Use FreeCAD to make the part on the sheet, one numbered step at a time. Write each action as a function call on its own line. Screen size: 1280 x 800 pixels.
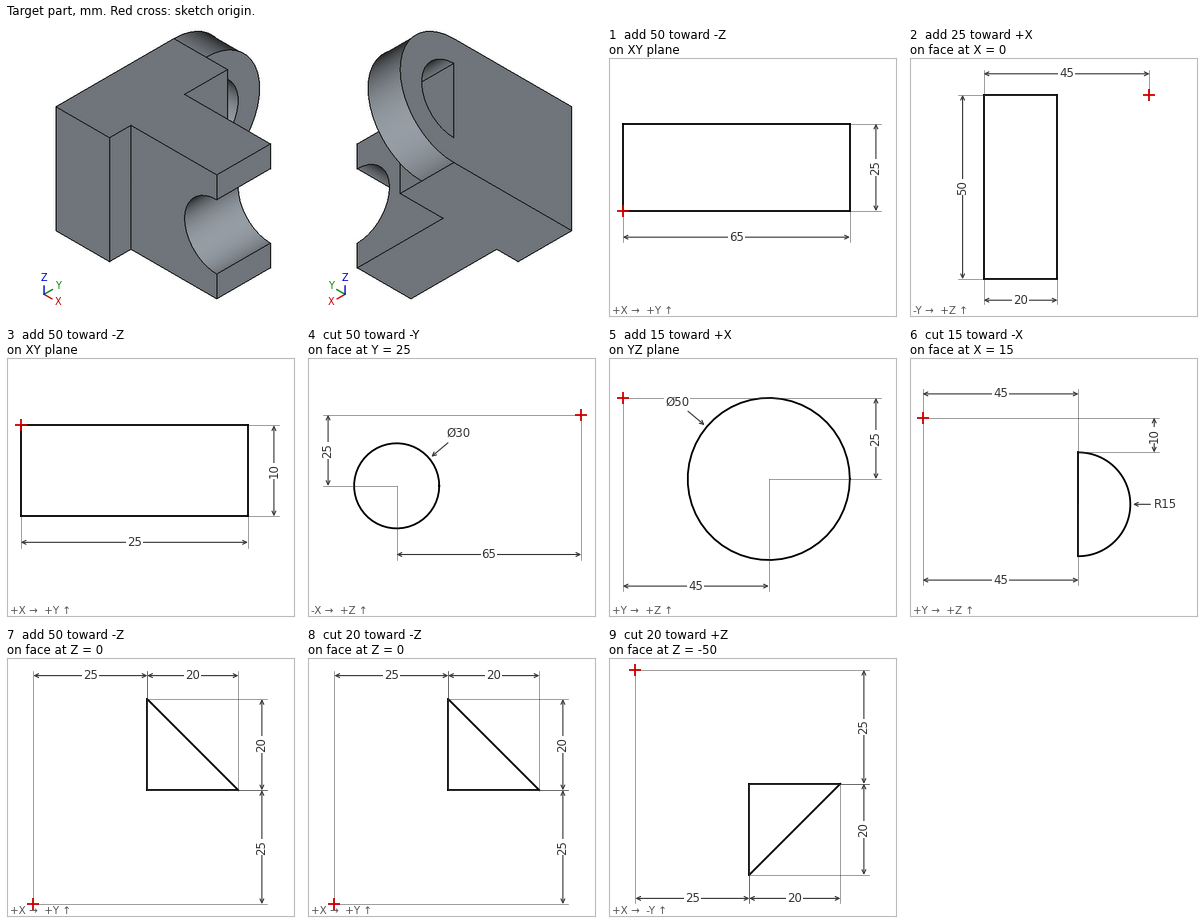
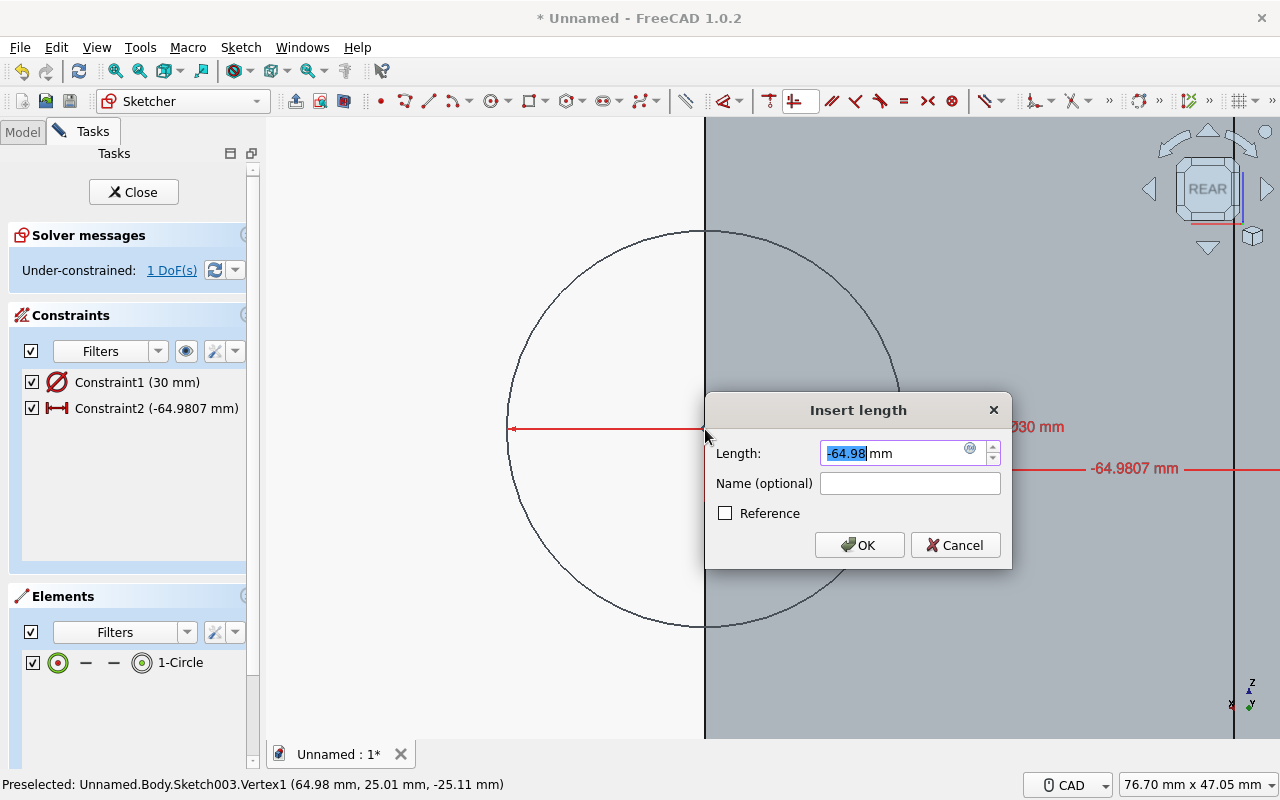
text(-65)
key(Return)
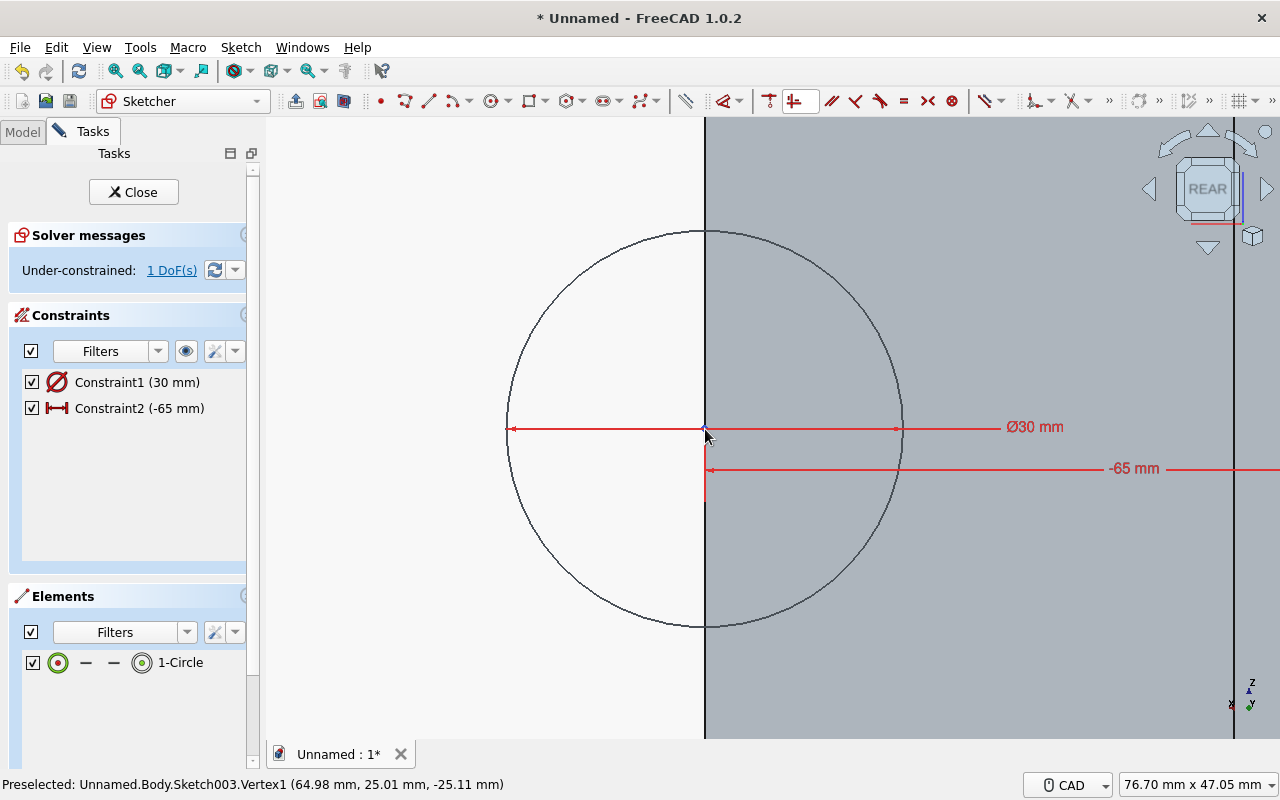
click(705, 429)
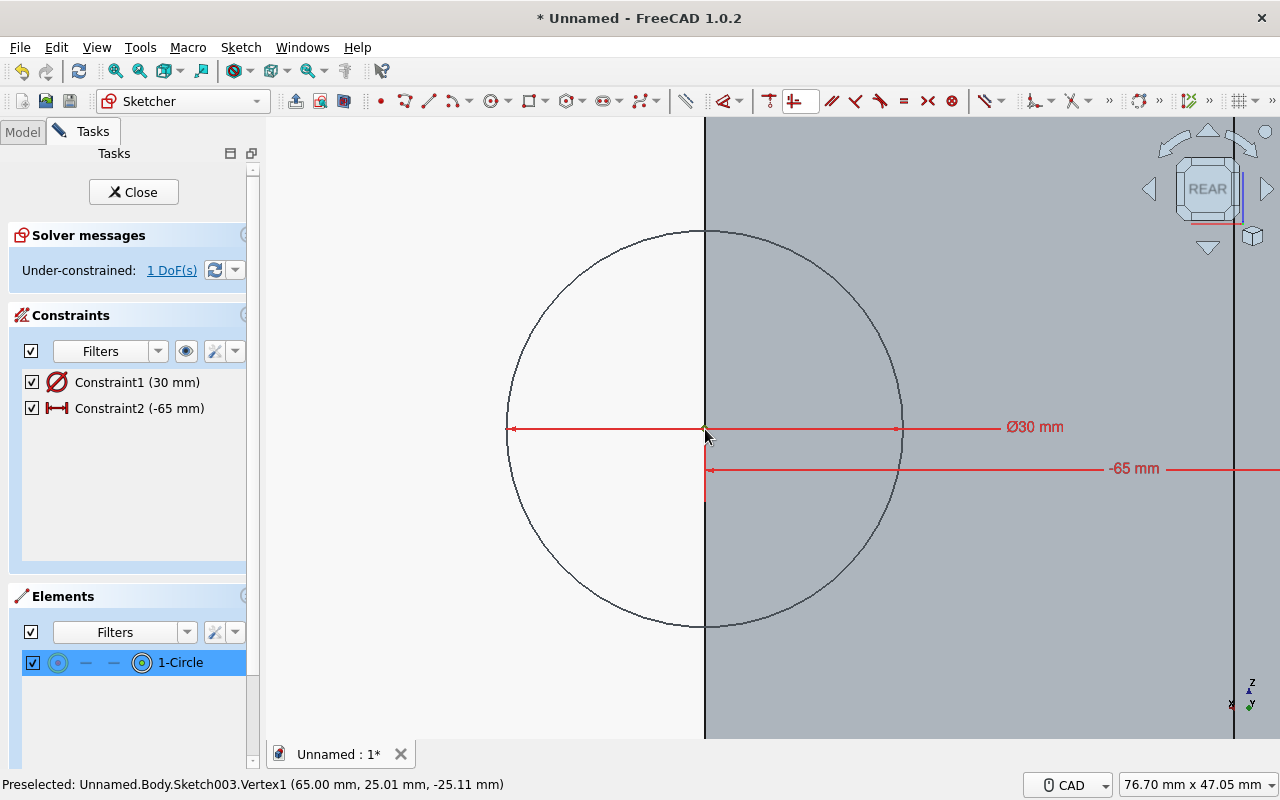
key(i)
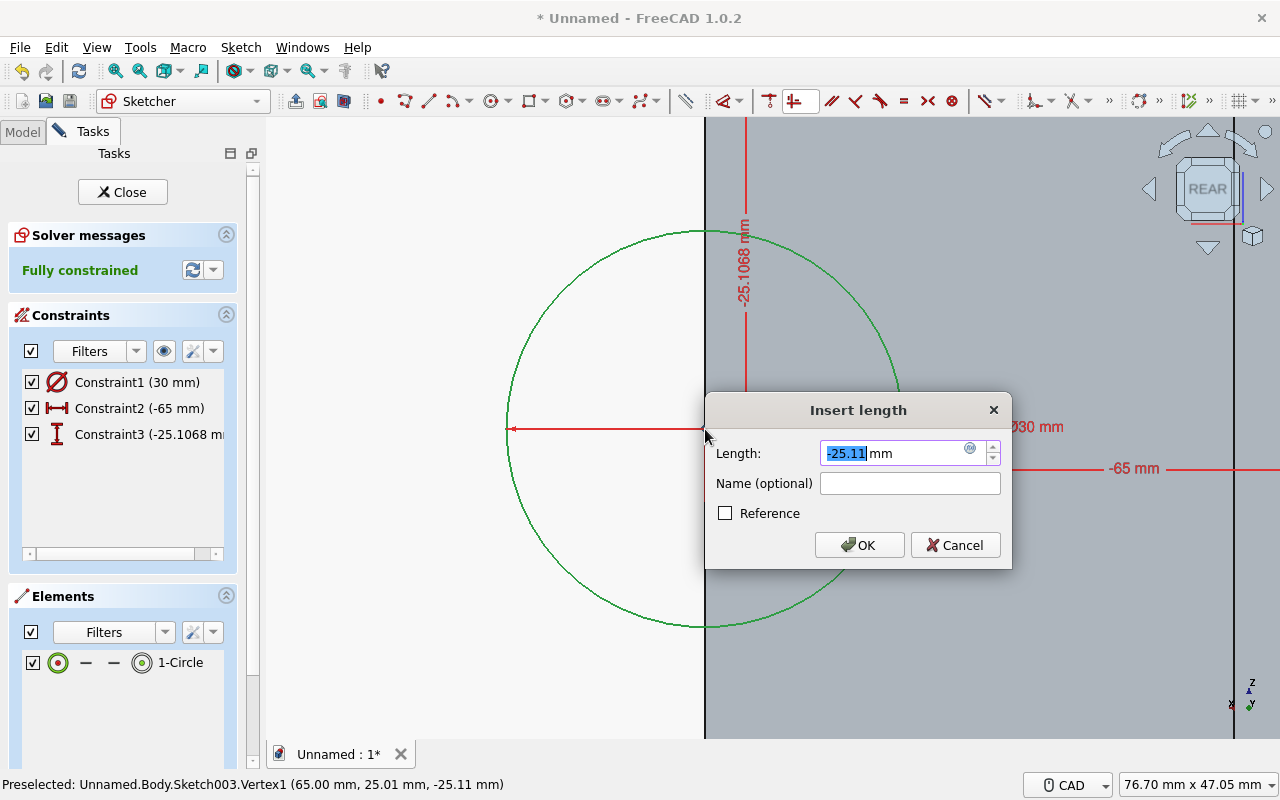
text(-25)
key(Return)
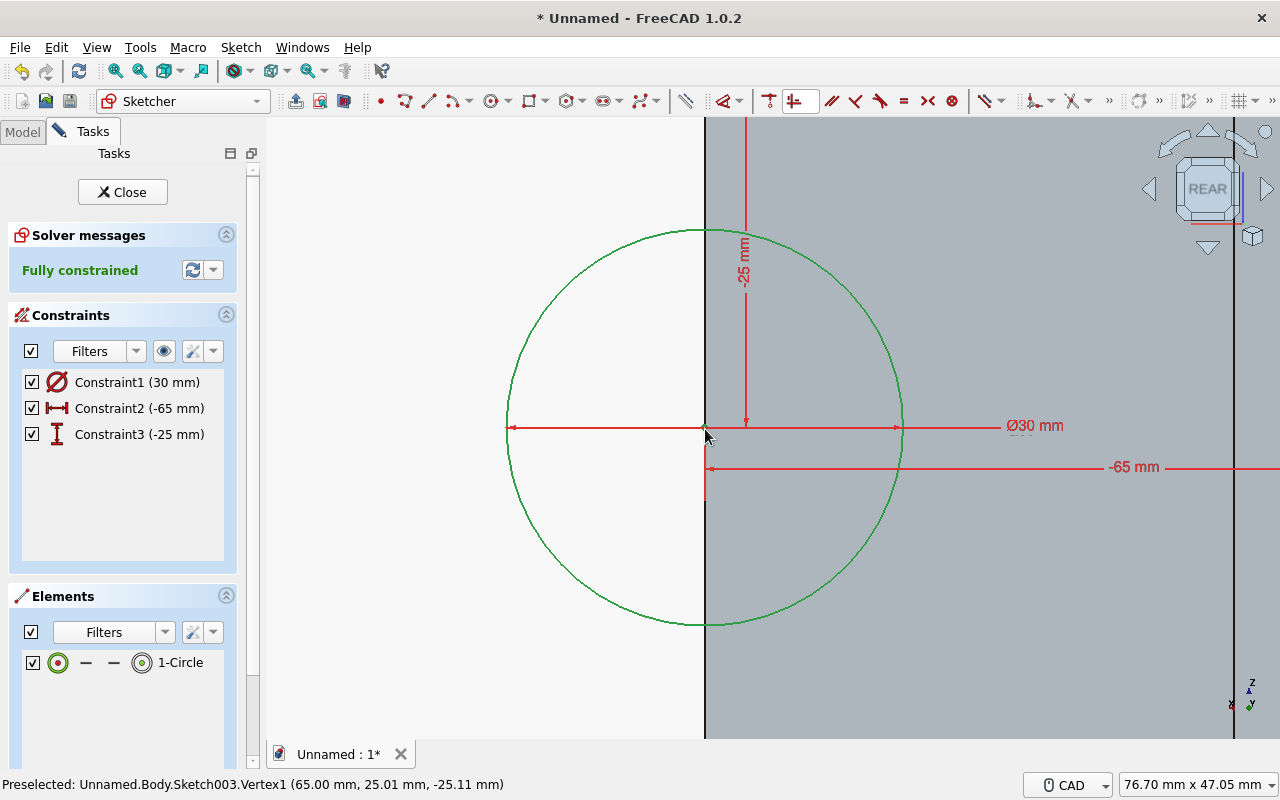
click(123, 192)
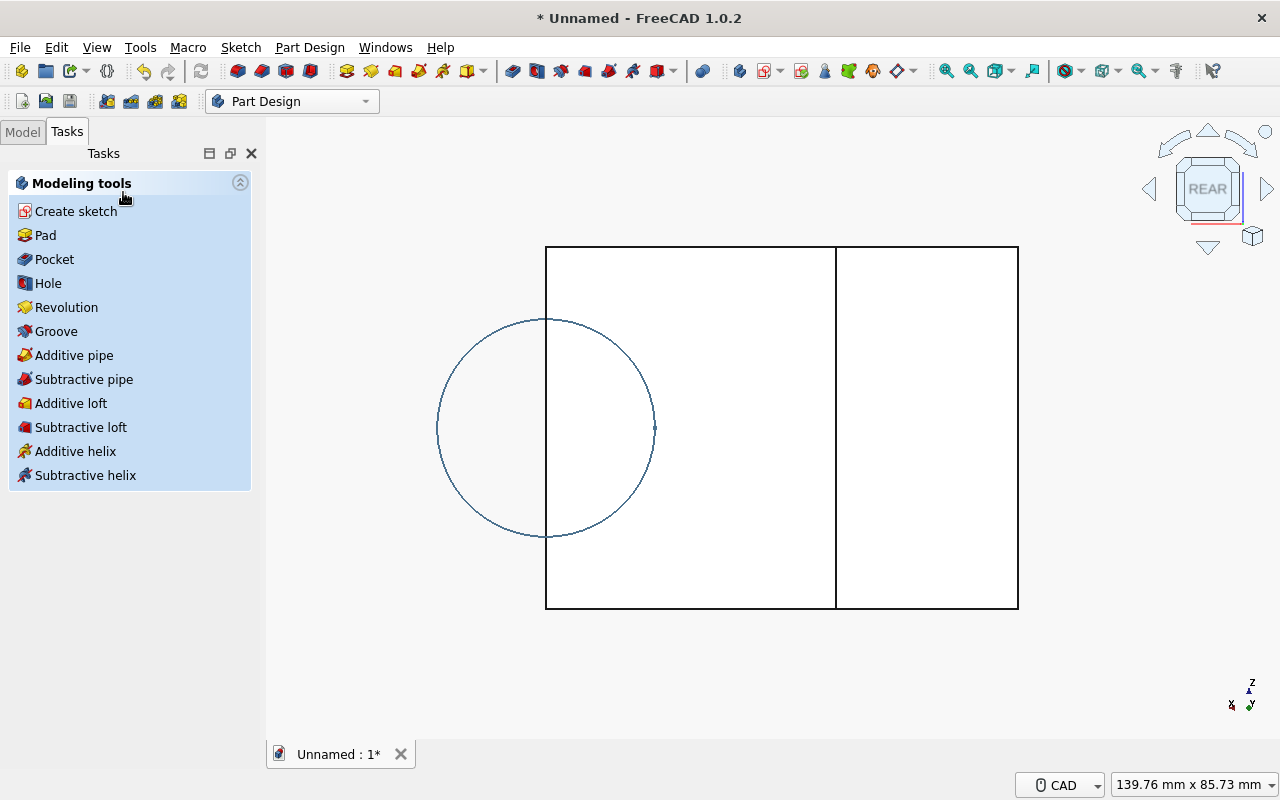
click(514, 72)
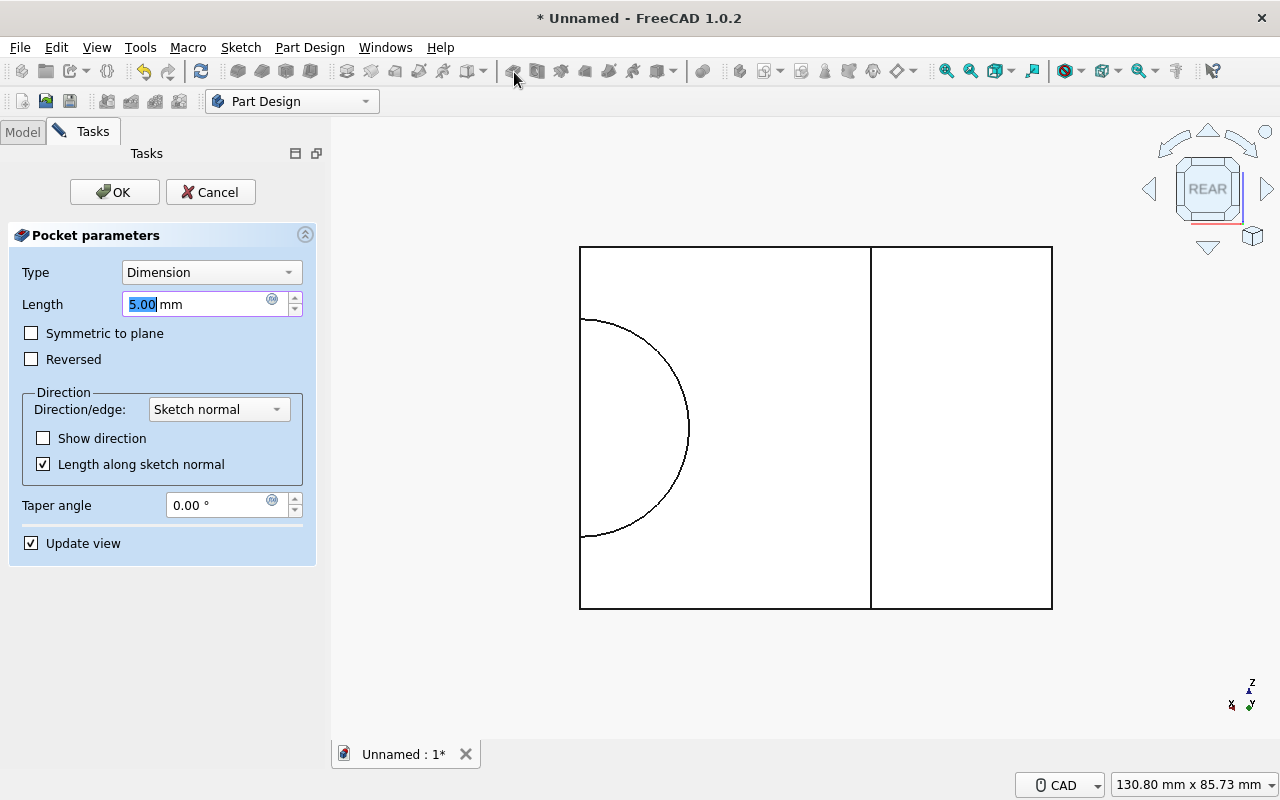
text(50)
key(Tab)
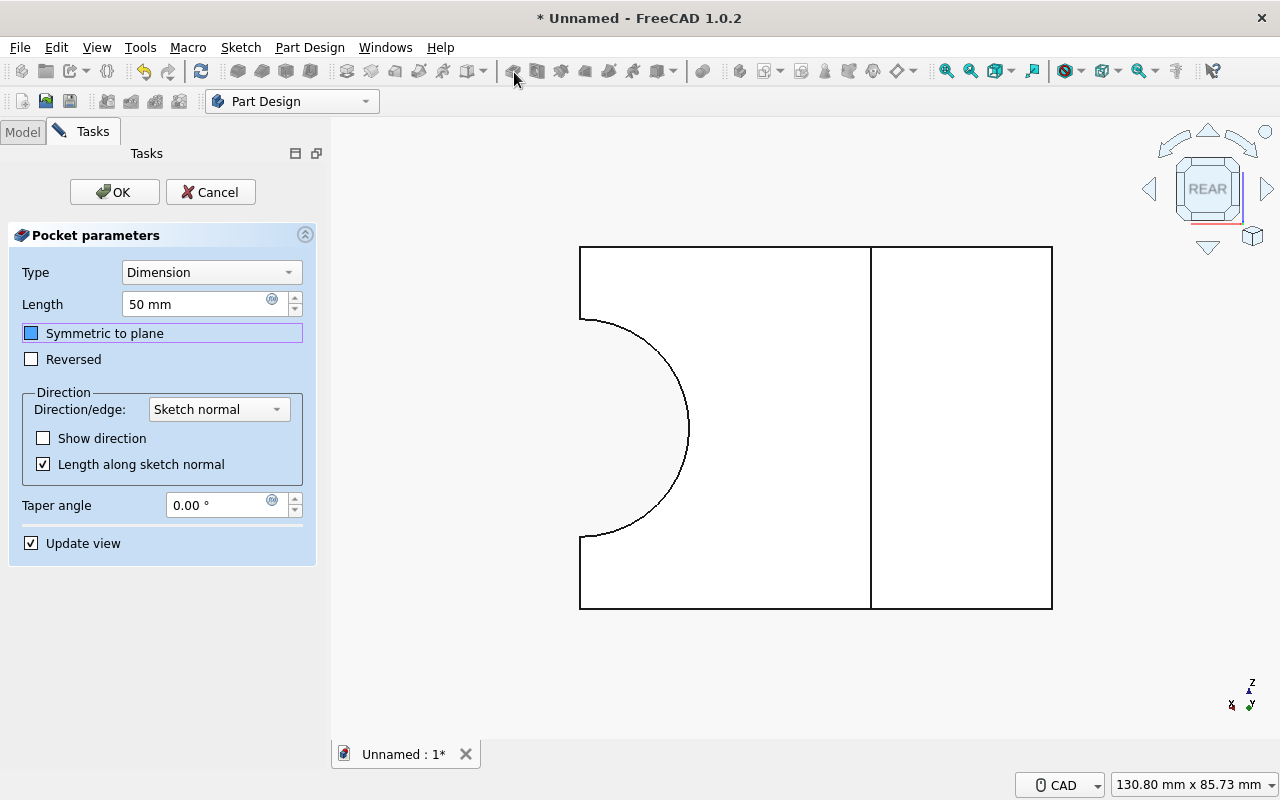
click(115, 192)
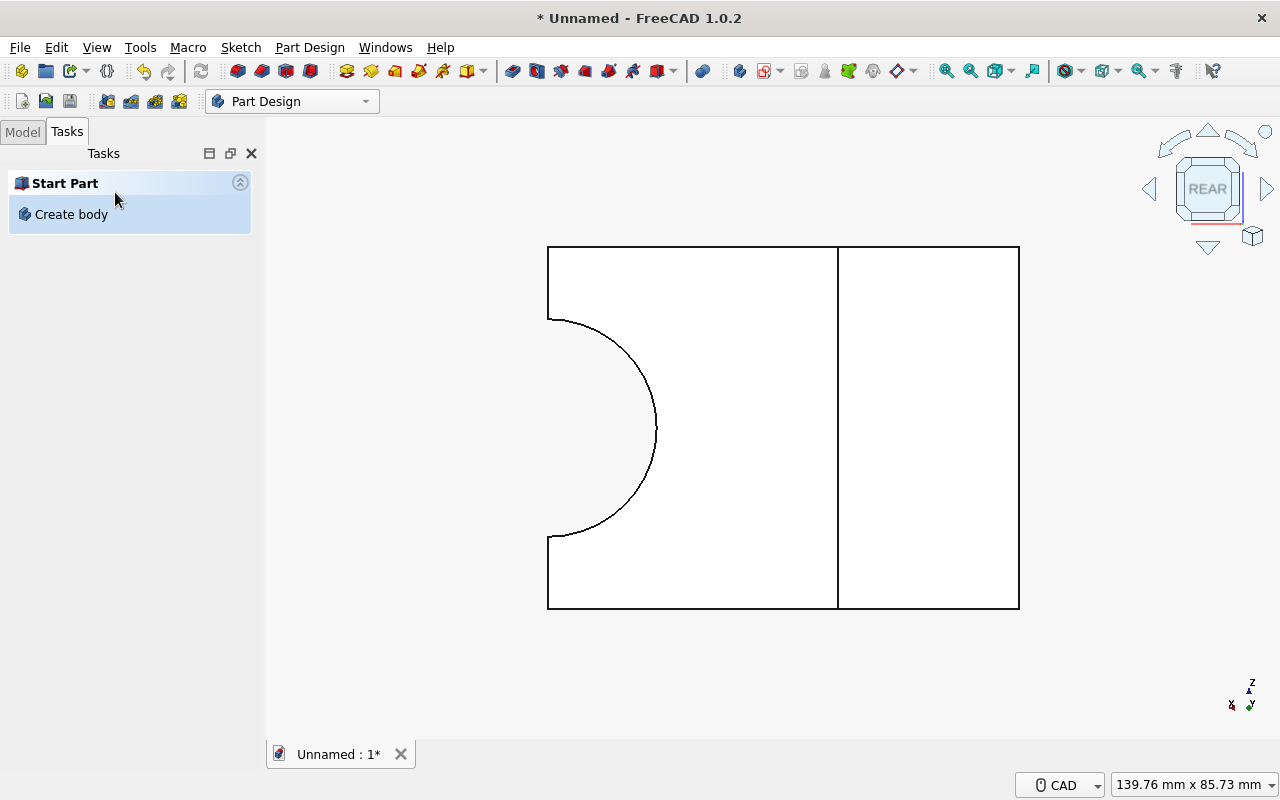
click(764, 72)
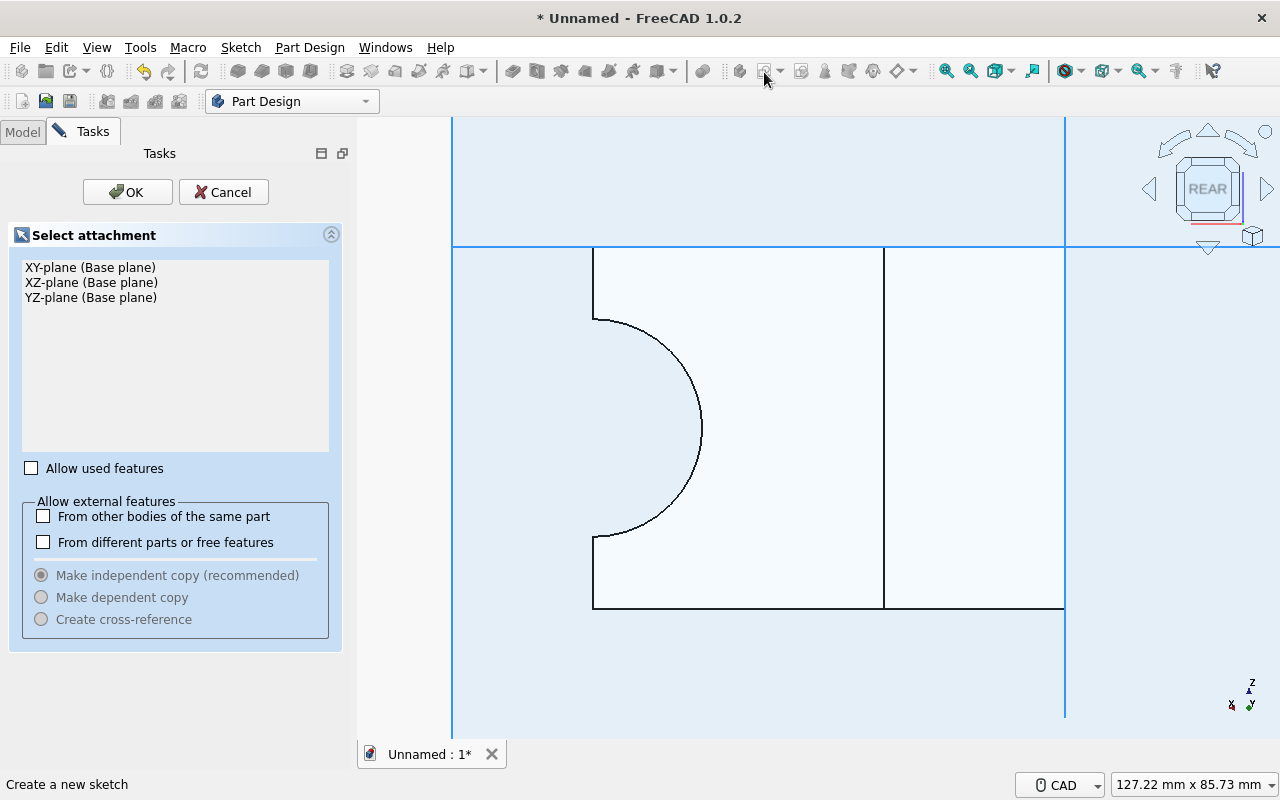
click(82, 298)